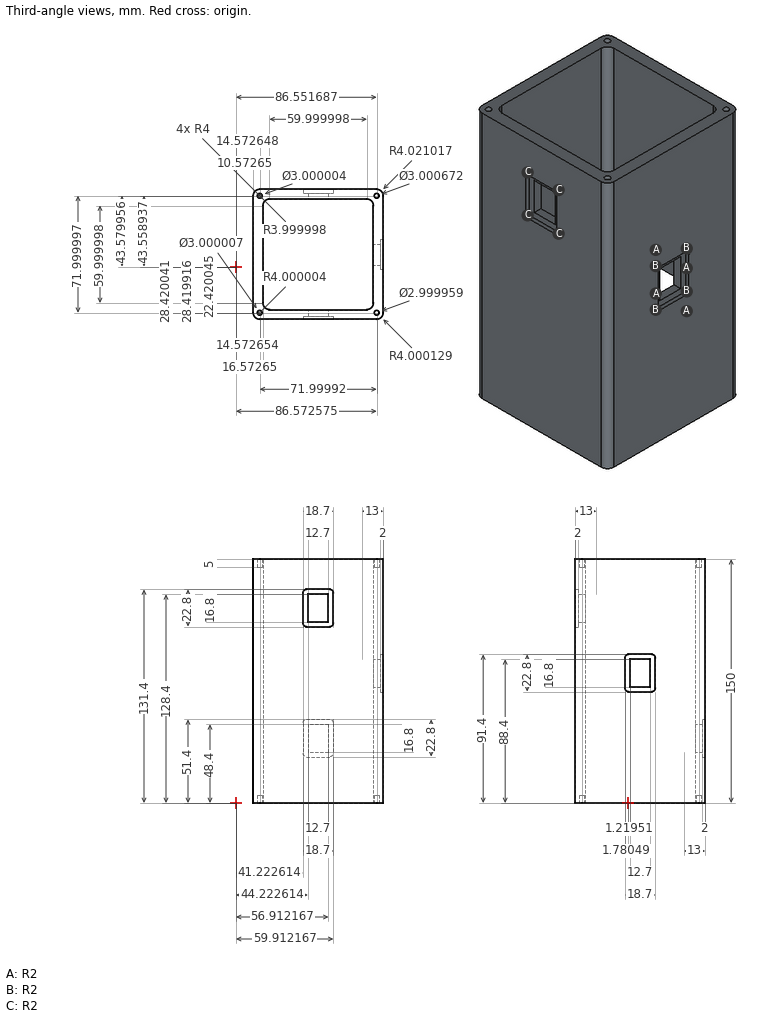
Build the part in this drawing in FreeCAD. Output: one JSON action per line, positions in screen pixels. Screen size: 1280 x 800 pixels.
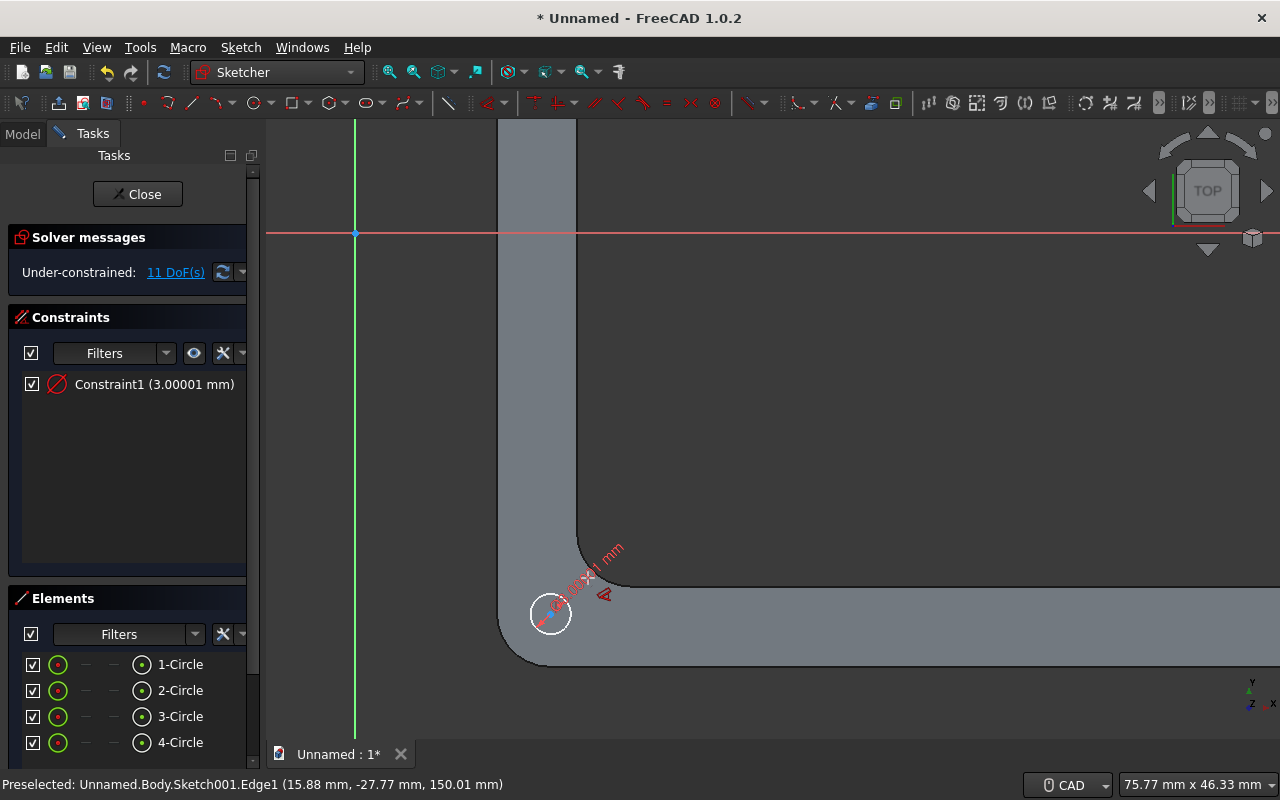
{"action": "scroll", "coordinate": [565, 602], "scroll_direction": "down", "scroll_amount": 5}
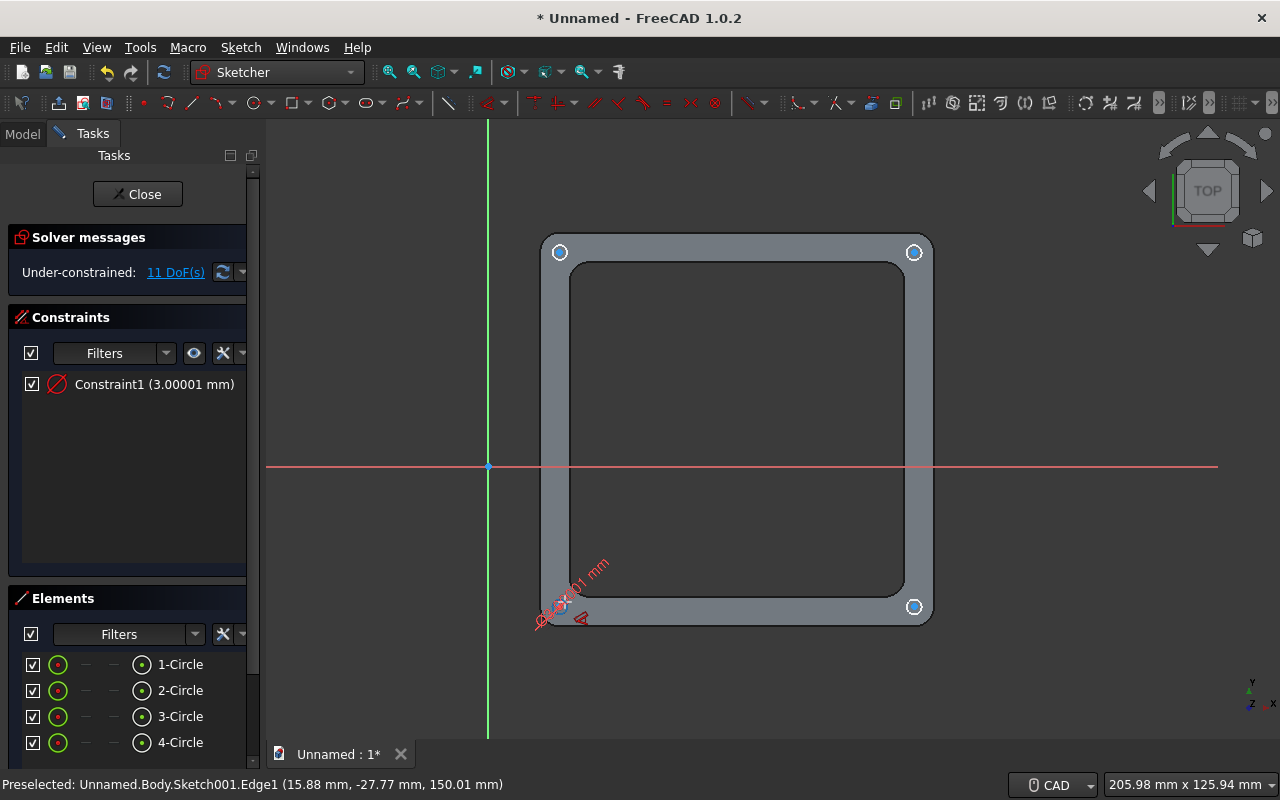
{"action": "scroll", "coordinate": [565, 247], "scroll_direction": "up", "scroll_amount": 5}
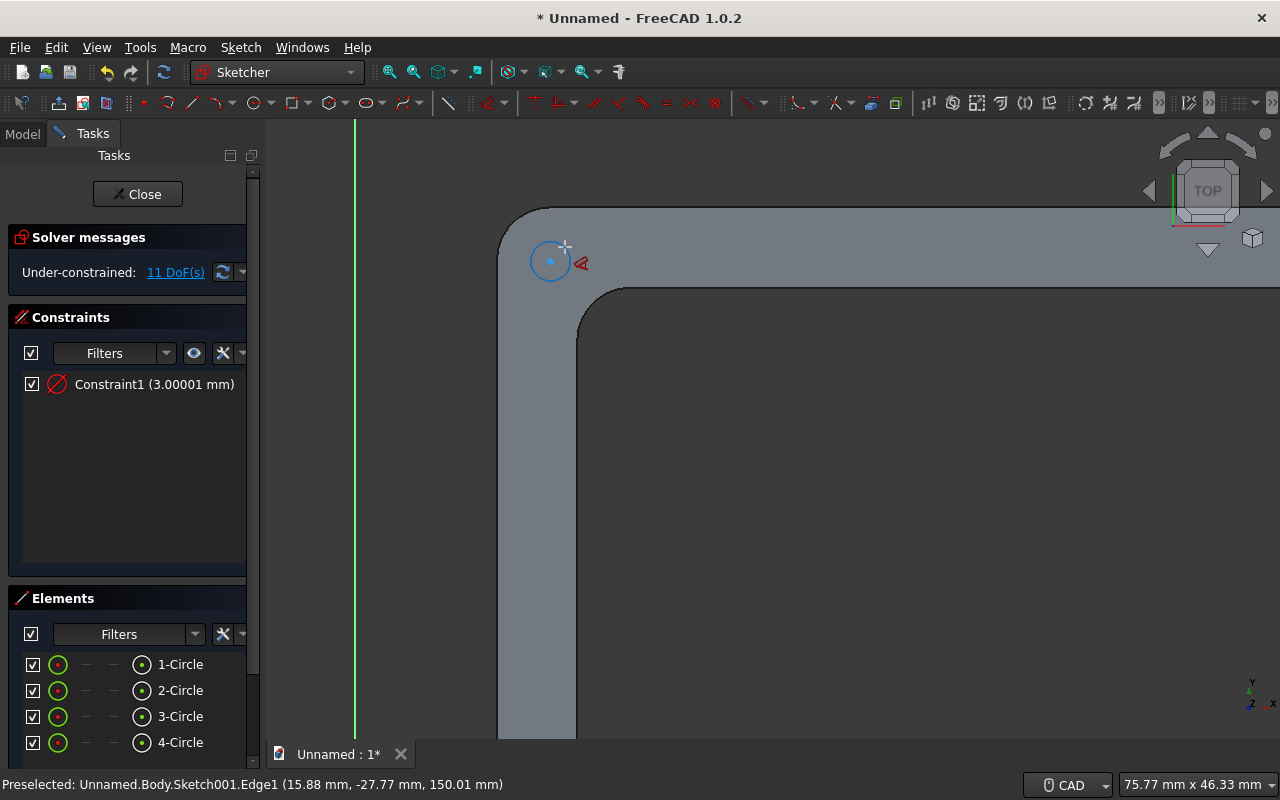
{"action": "left_click", "coordinate": [565, 248]}
{"action": "left_click", "coordinate": [588, 226]}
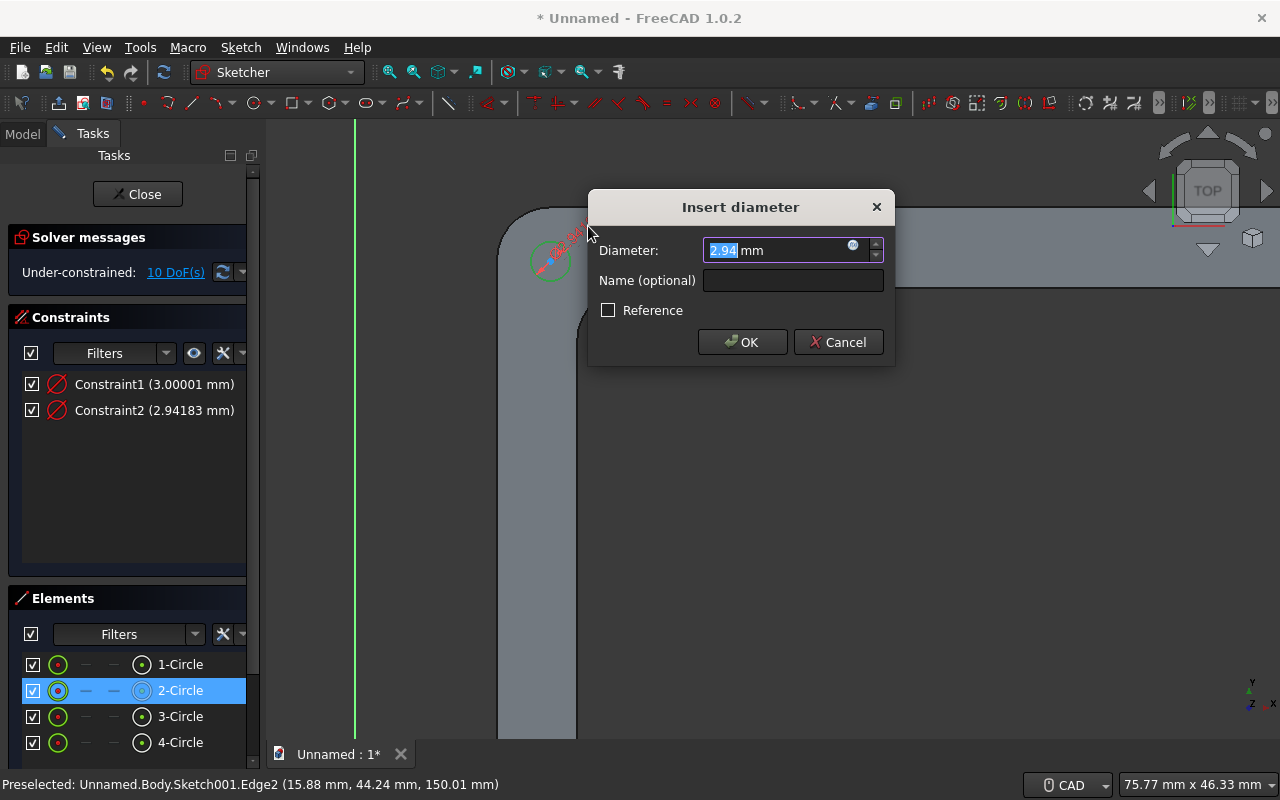
{"action": "type", "text": "3.000004"}
{"action": "key", "text": "Return"}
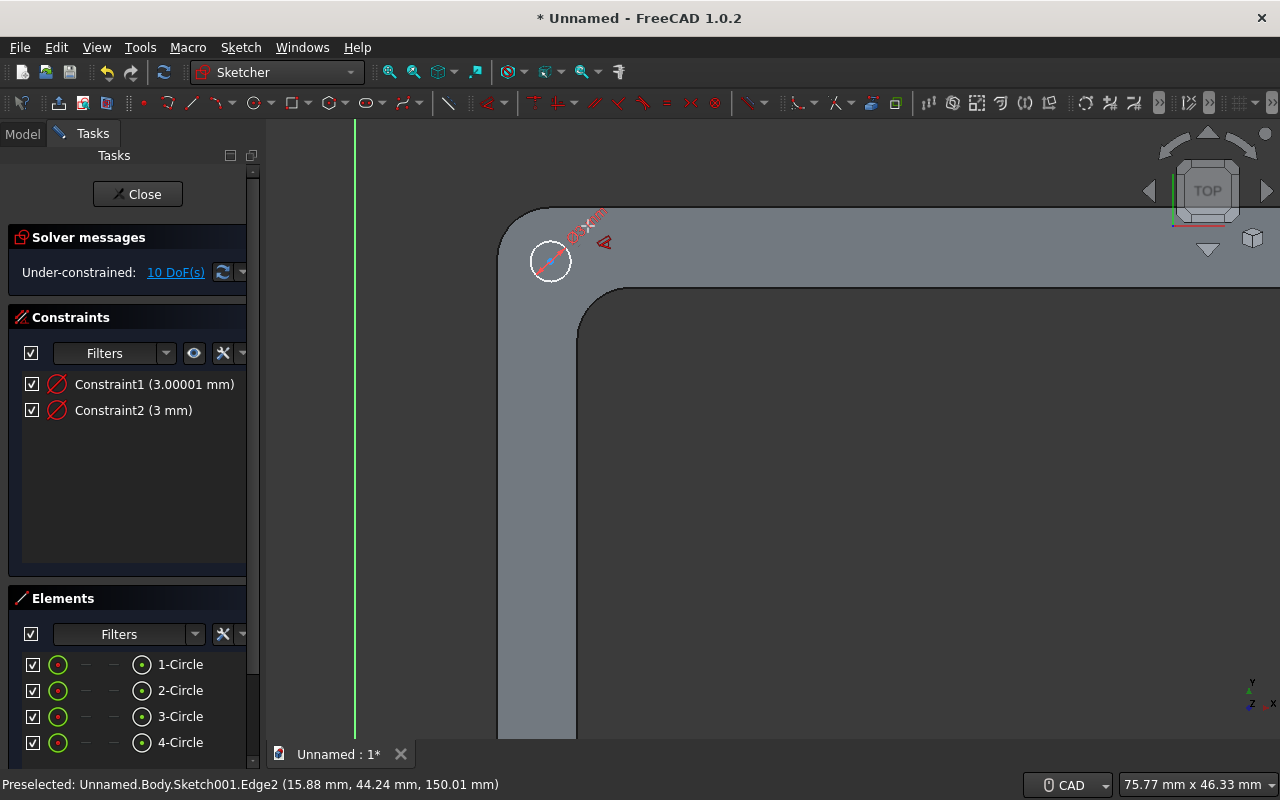
{"action": "scroll", "coordinate": [565, 246], "scroll_direction": "down", "scroll_amount": 5}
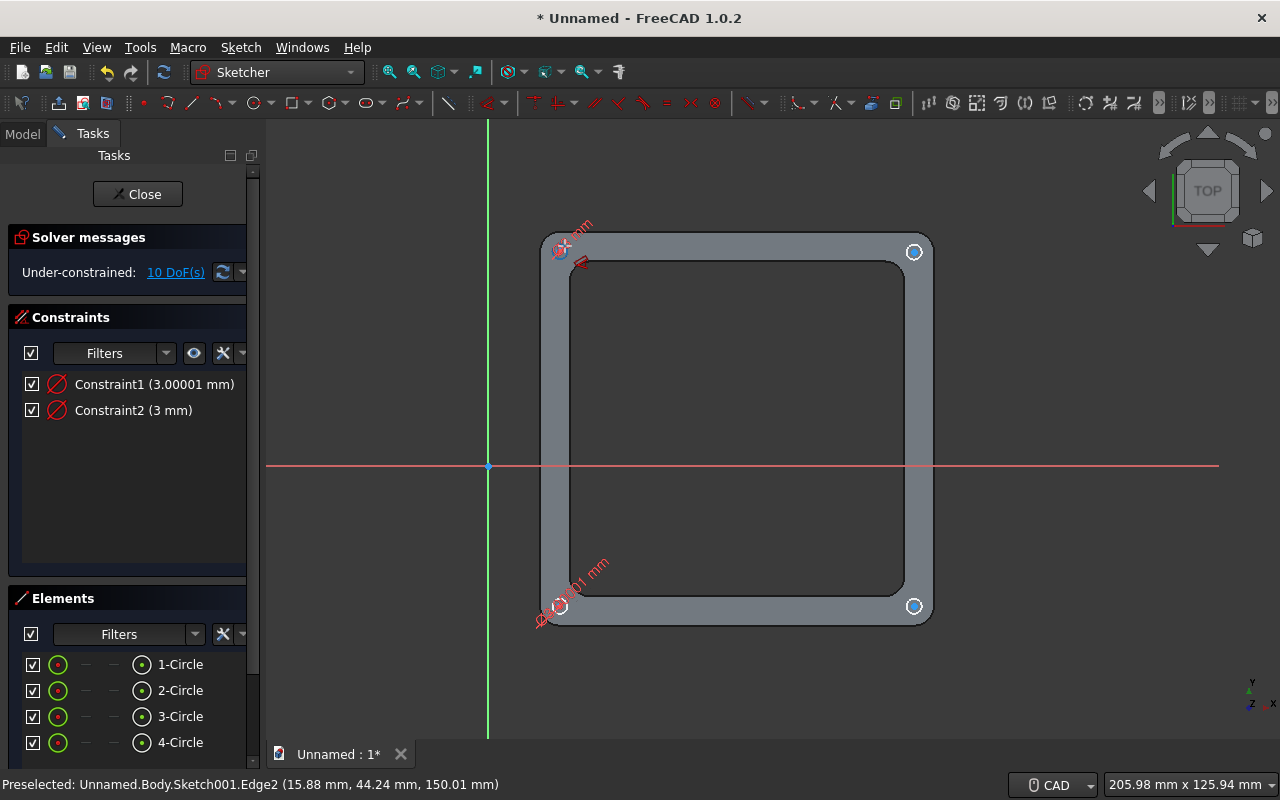
{"action": "scroll", "coordinate": [919, 247], "scroll_direction": "up", "scroll_amount": 5}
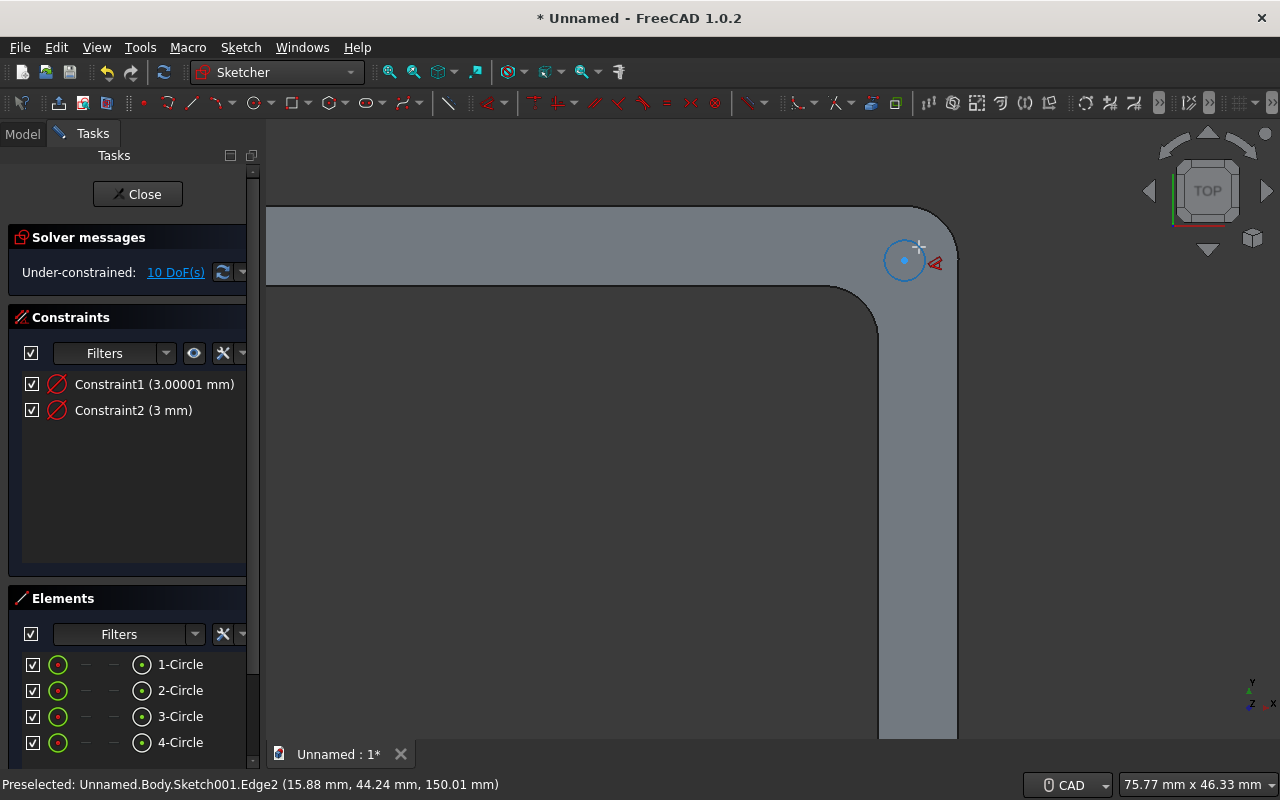
{"action": "left_click", "coordinate": [919, 246]}
{"action": "left_click", "coordinate": [941, 223]}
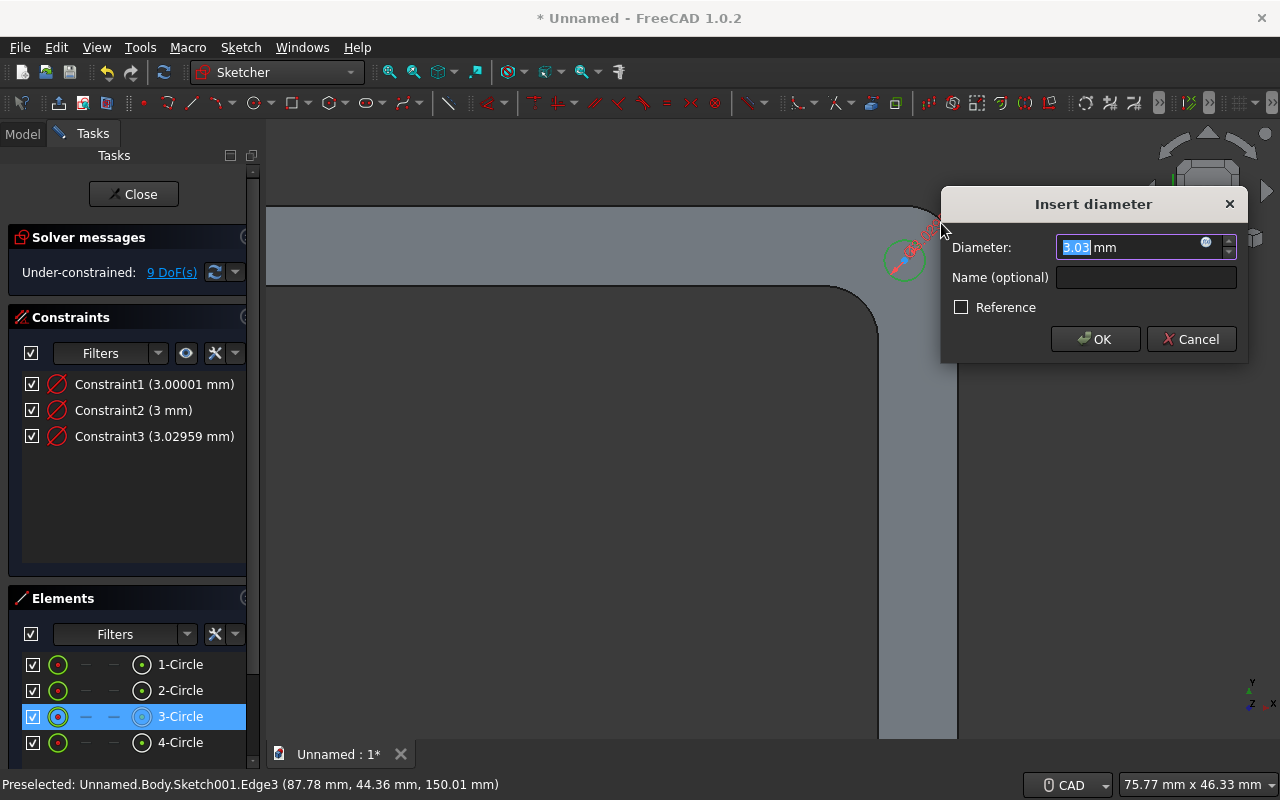
{"action": "type", "text": "3.000672"}
{"action": "key", "text": "Return"}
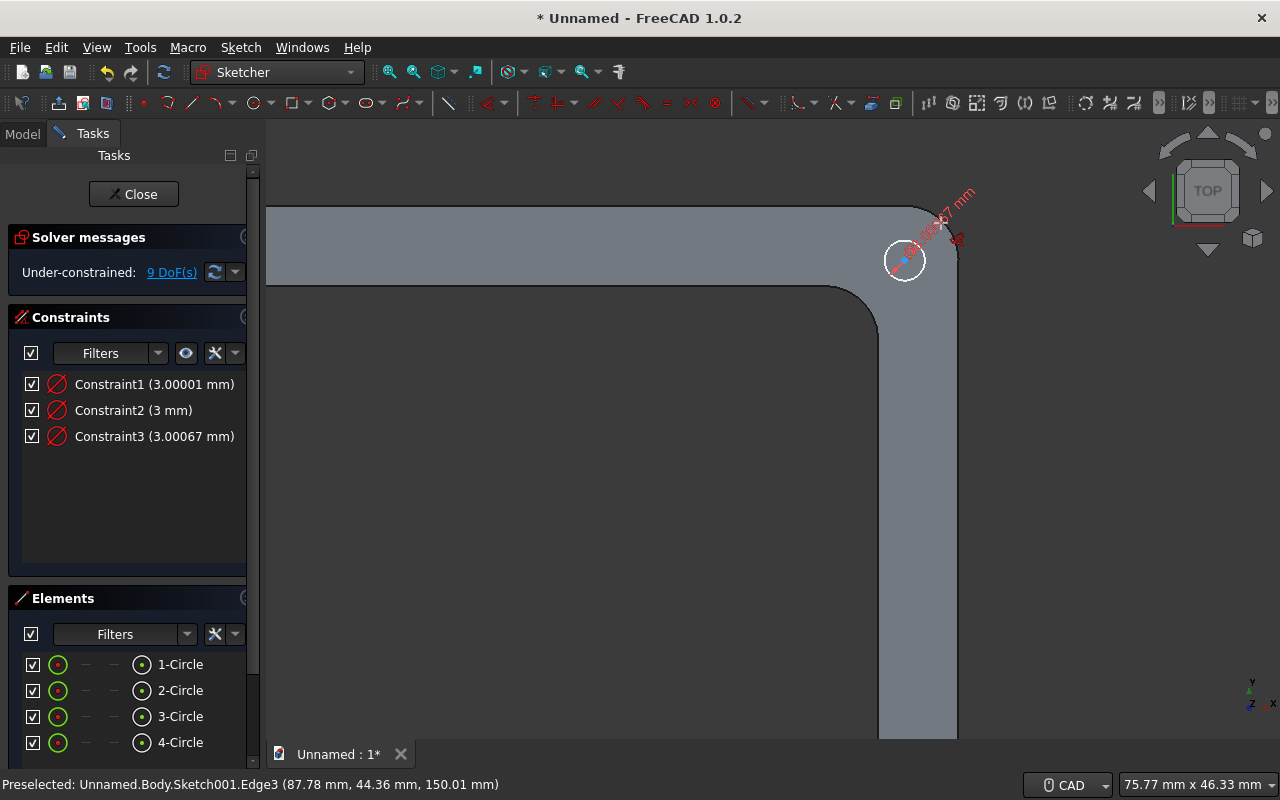
{"action": "scroll", "coordinate": [919, 247], "scroll_direction": "down", "scroll_amount": 5}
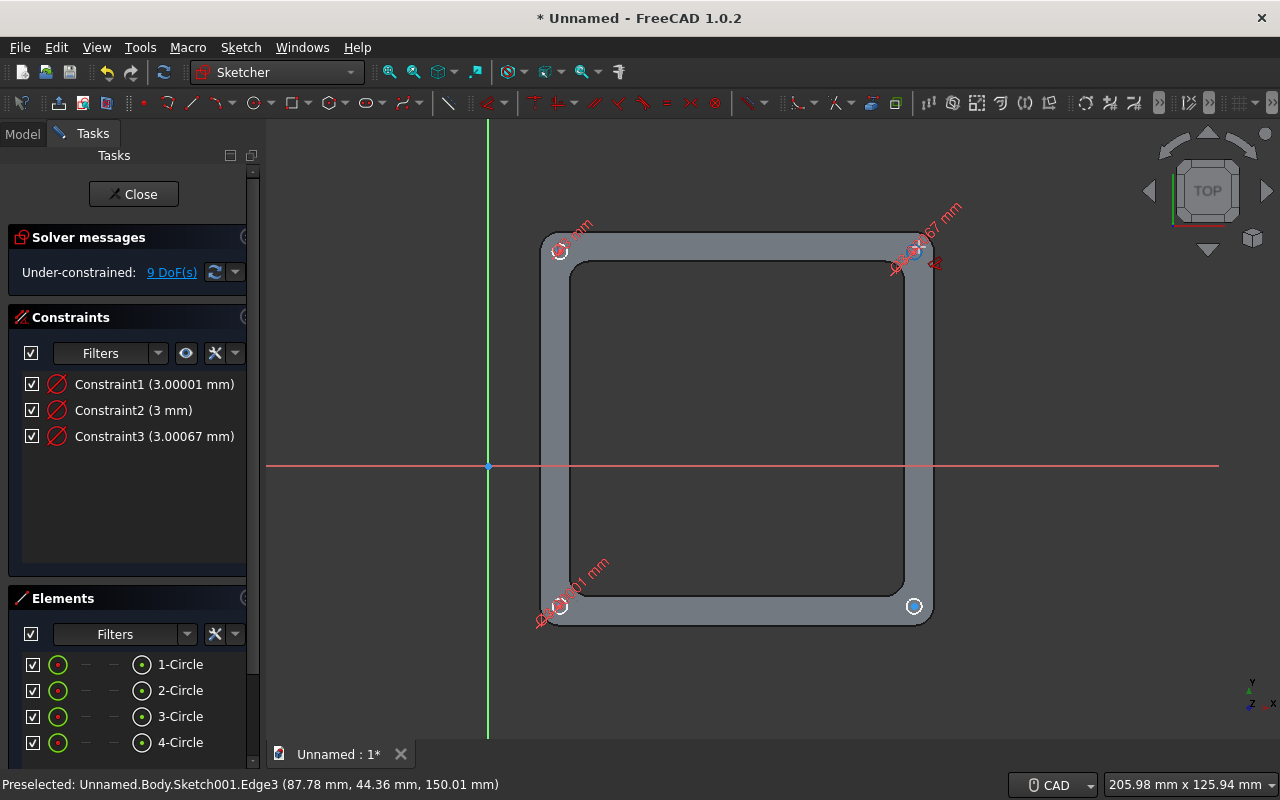
{"action": "scroll", "coordinate": [919, 601], "scroll_direction": "up", "scroll_amount": 5}